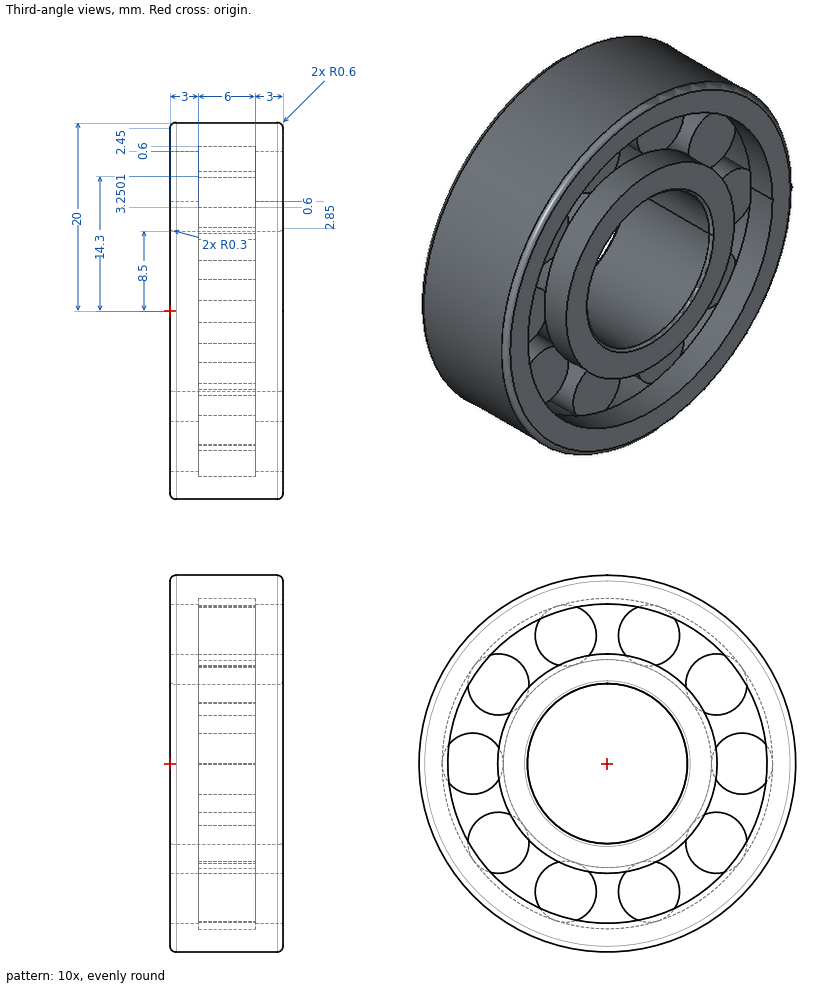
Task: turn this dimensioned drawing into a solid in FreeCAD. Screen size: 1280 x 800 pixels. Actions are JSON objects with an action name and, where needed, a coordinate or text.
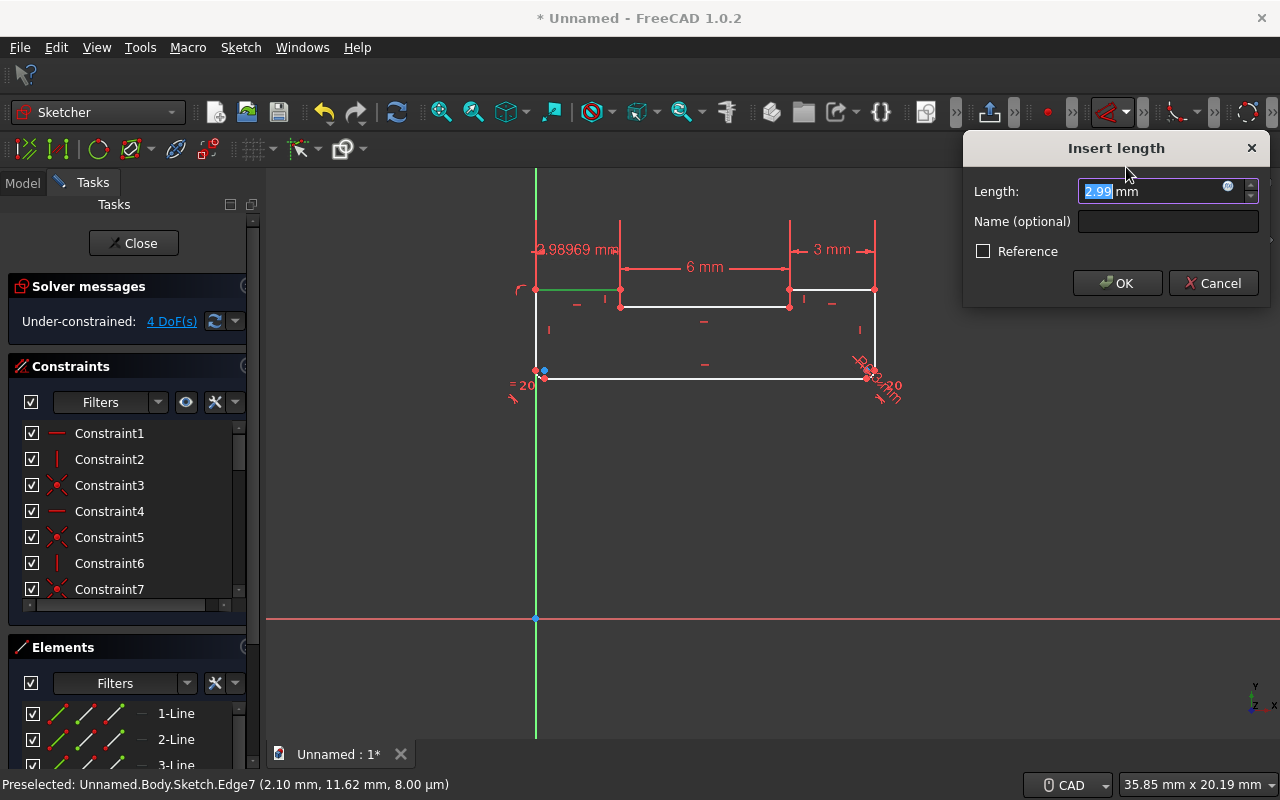
{"action": "type", "text": "3"}
{"action": "key", "text": "Return"}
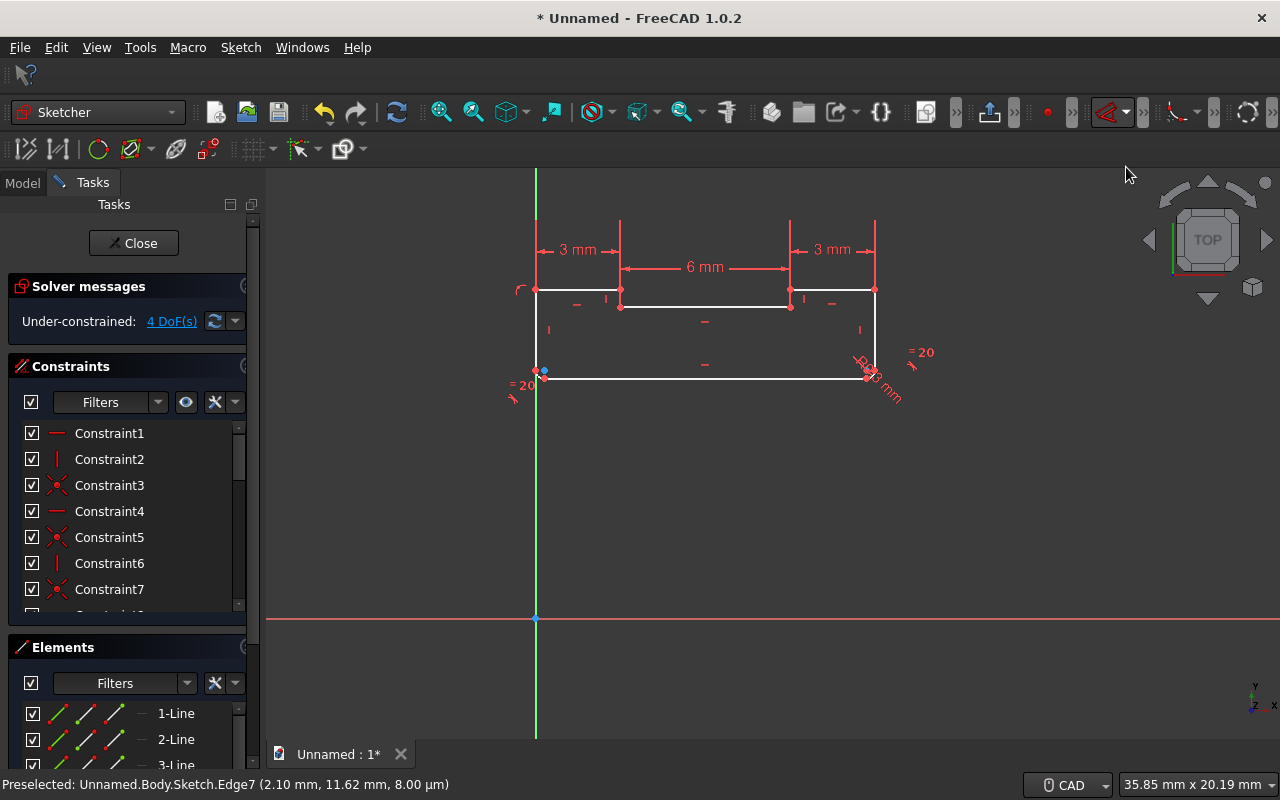
{"action": "scroll", "coordinate": [790, 298], "scroll_direction": "up", "scroll_amount": 5}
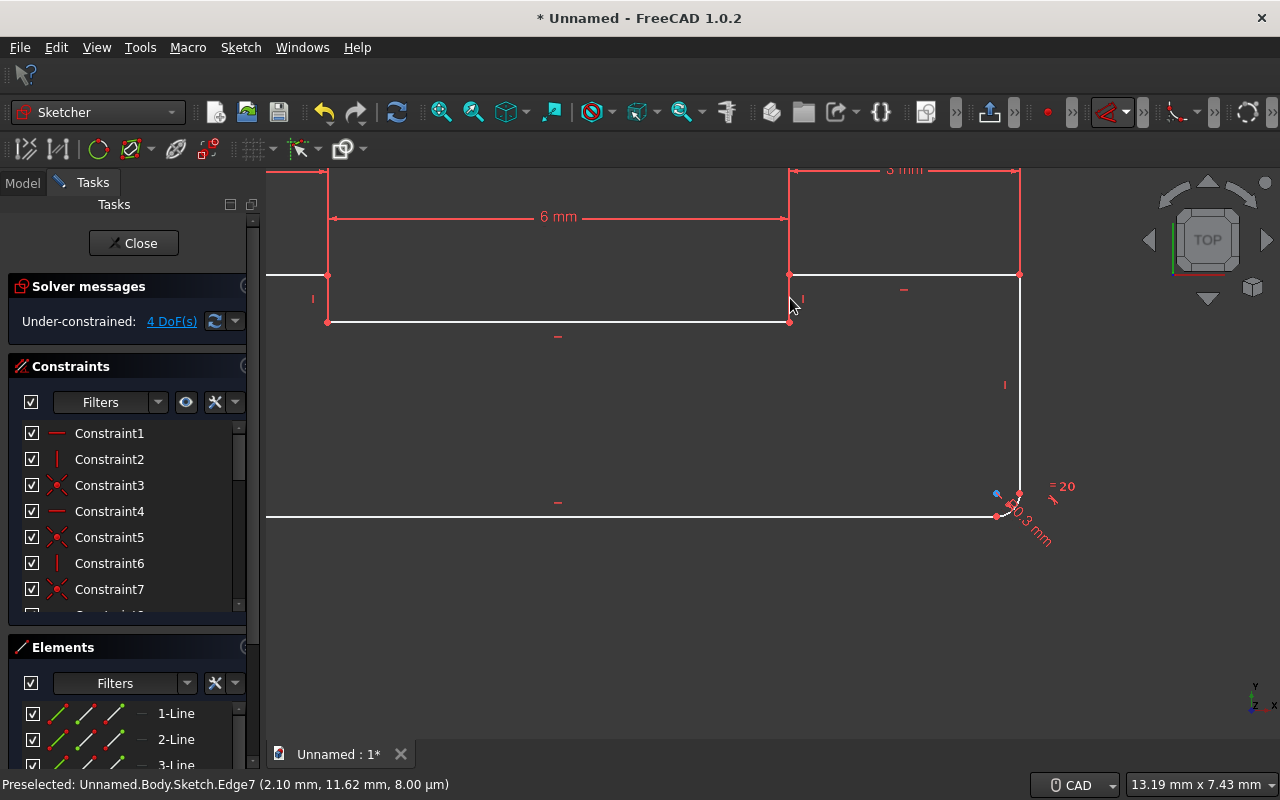
{"action": "left_click", "coordinate": [789, 298]}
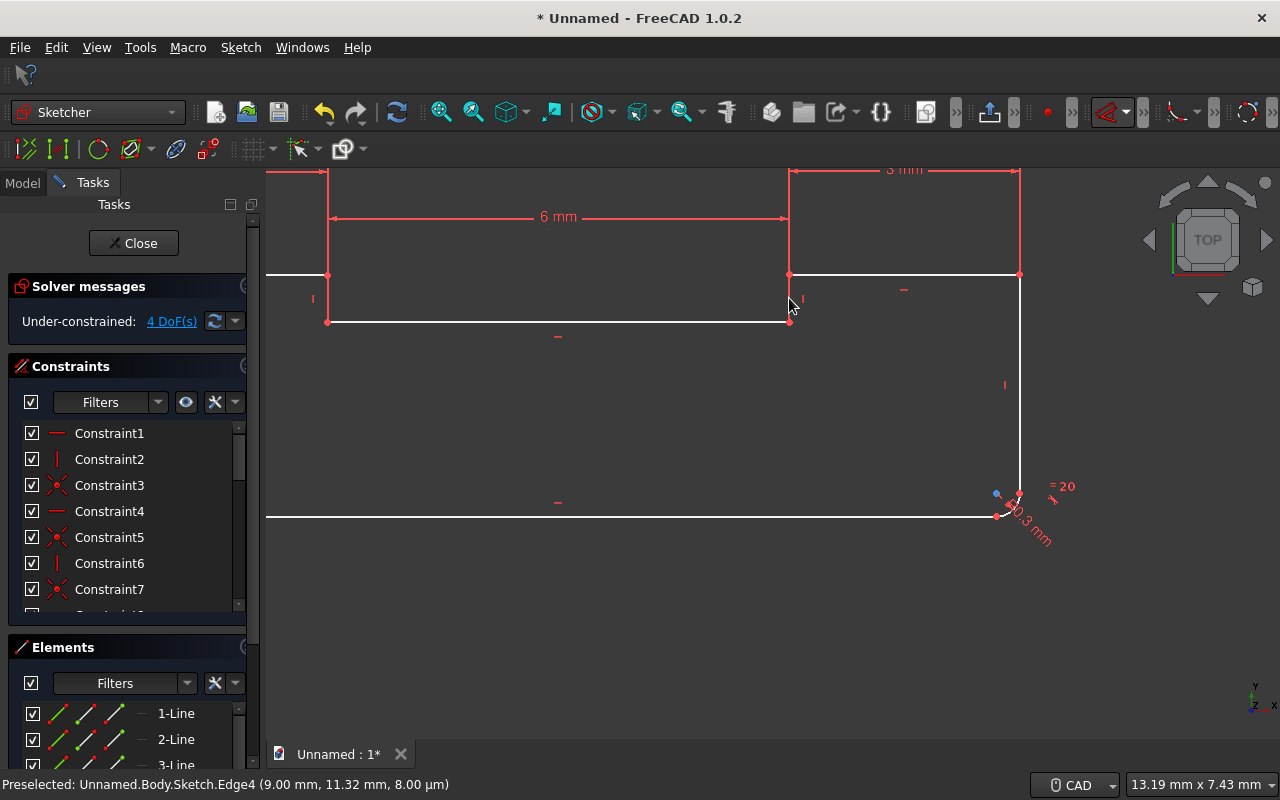
{"action": "left_click", "coordinate": [1128, 112]}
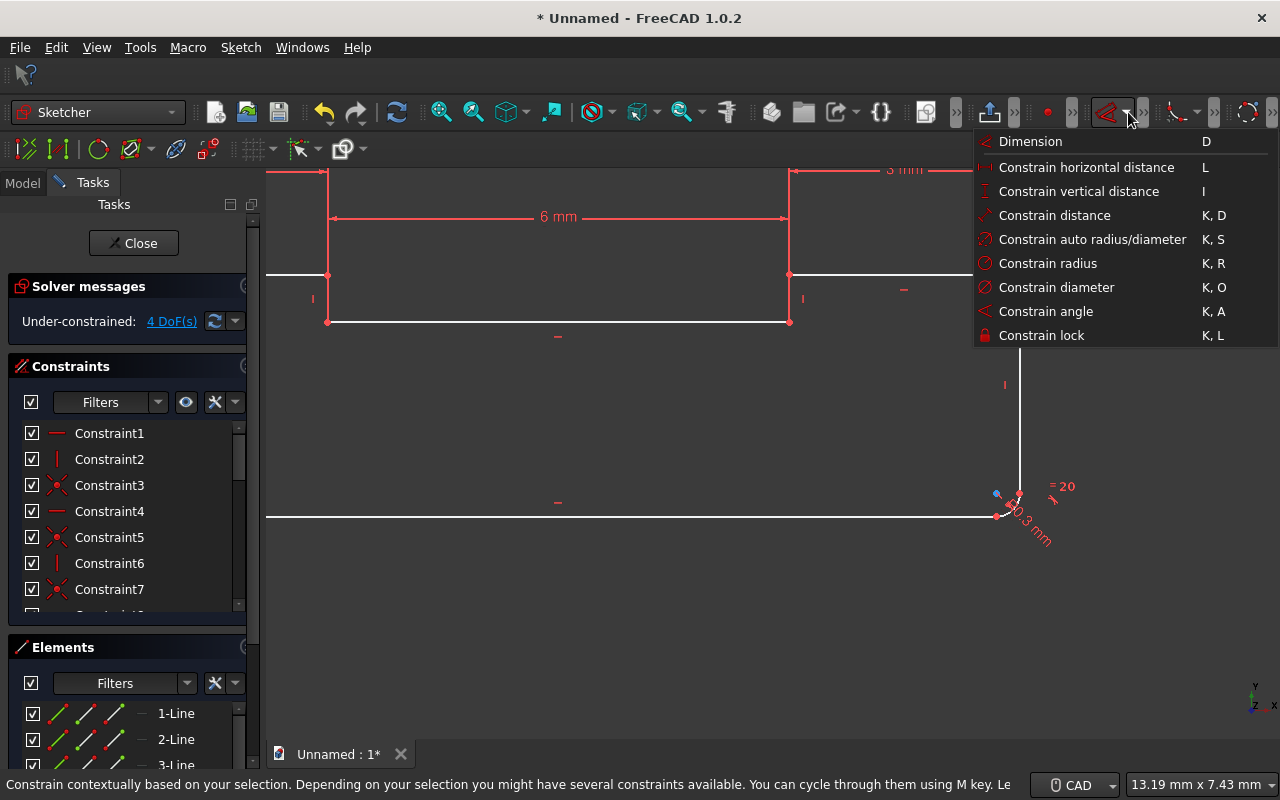
{"action": "left_click", "coordinate": [1126, 191]}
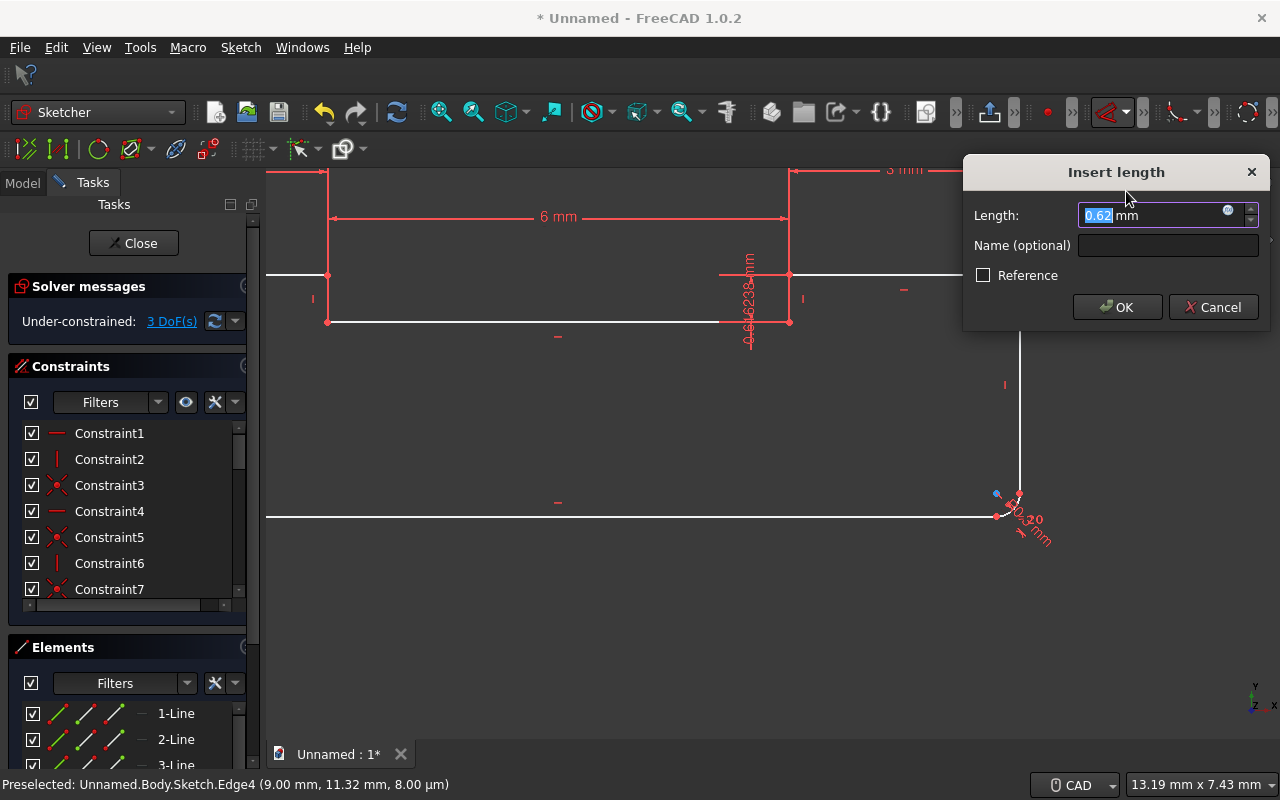
{"action": "type", "text": "0.6"}
{"action": "key", "text": "Return"}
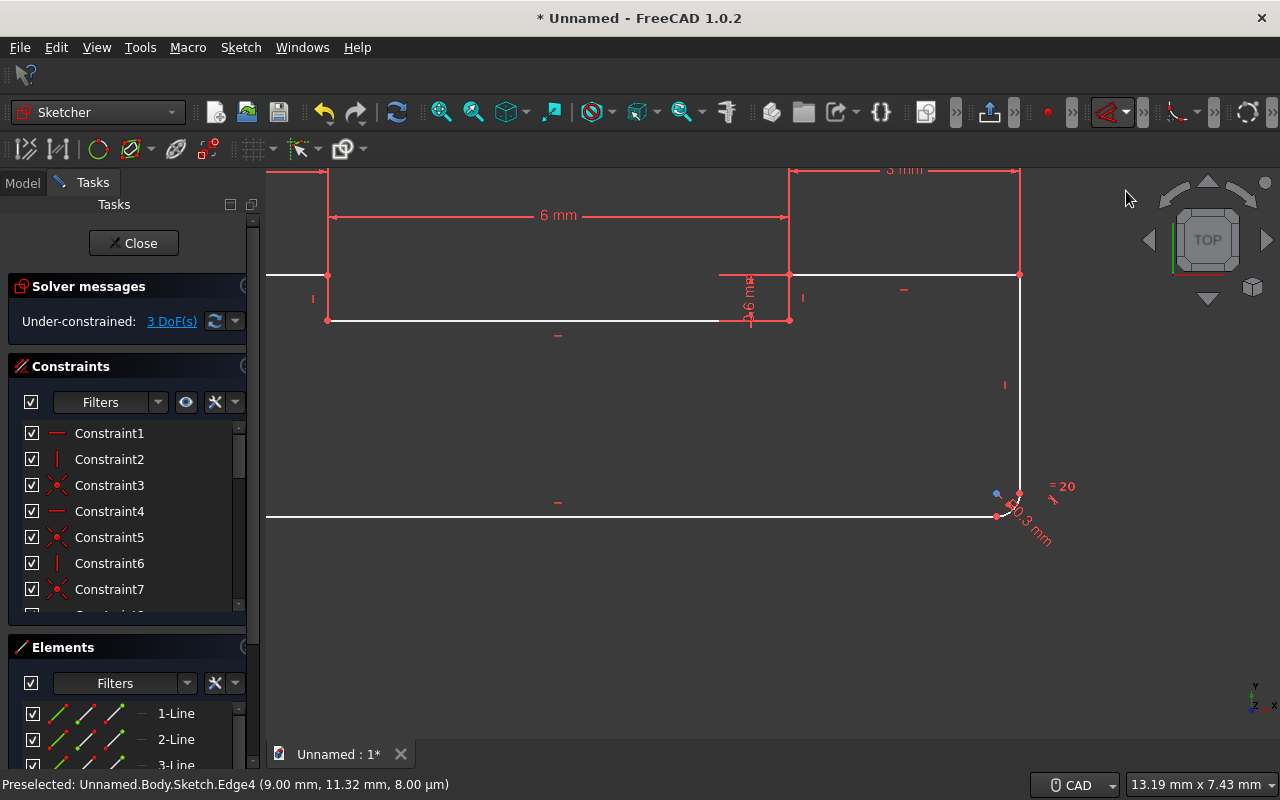
{"action": "left_click", "coordinate": [328, 307]}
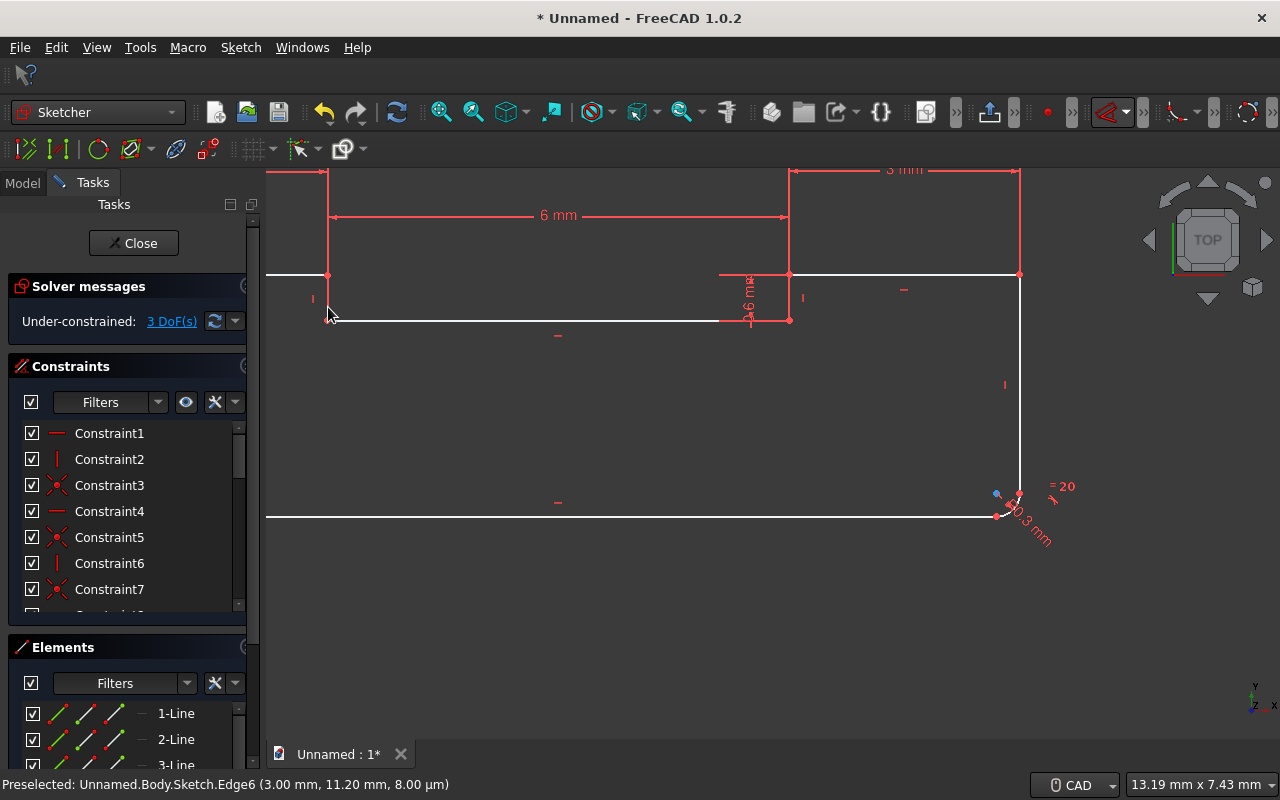
{"action": "left_click", "coordinate": [1128, 112]}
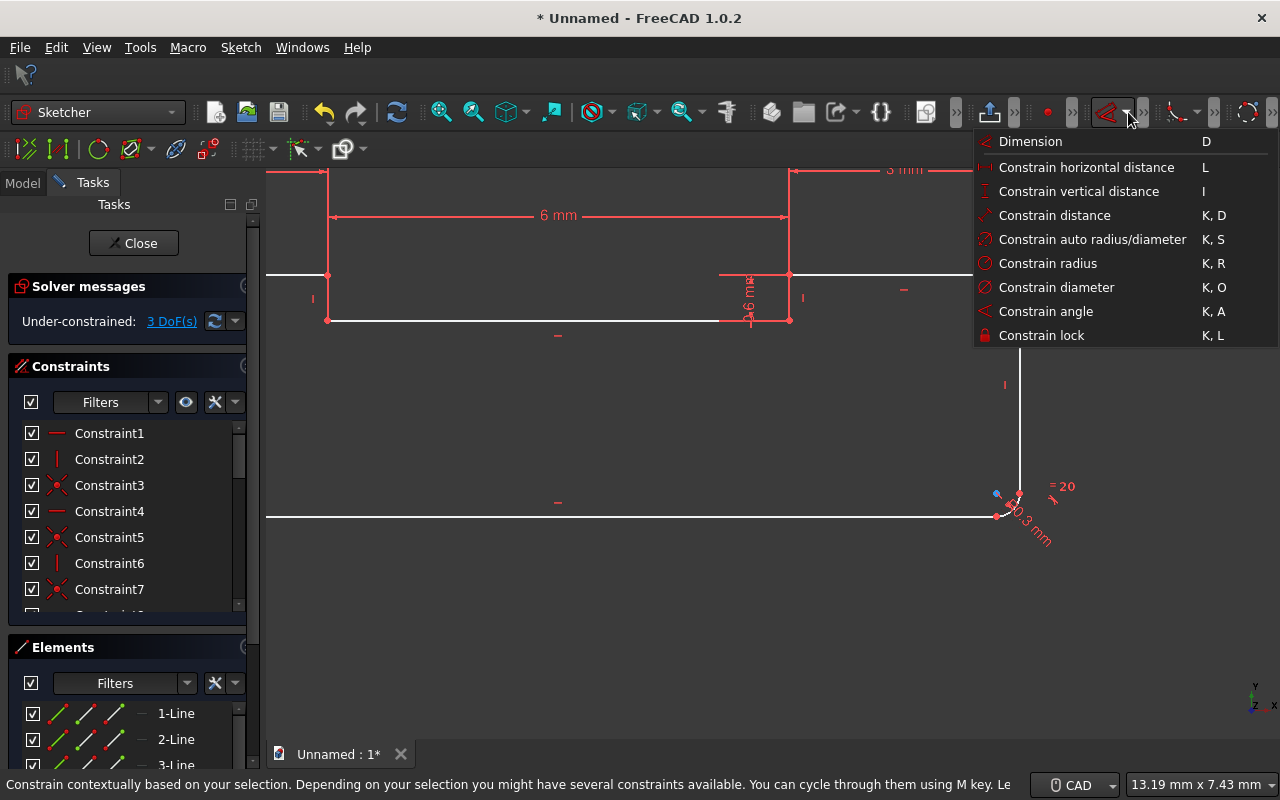
{"action": "left_click", "coordinate": [1126, 191]}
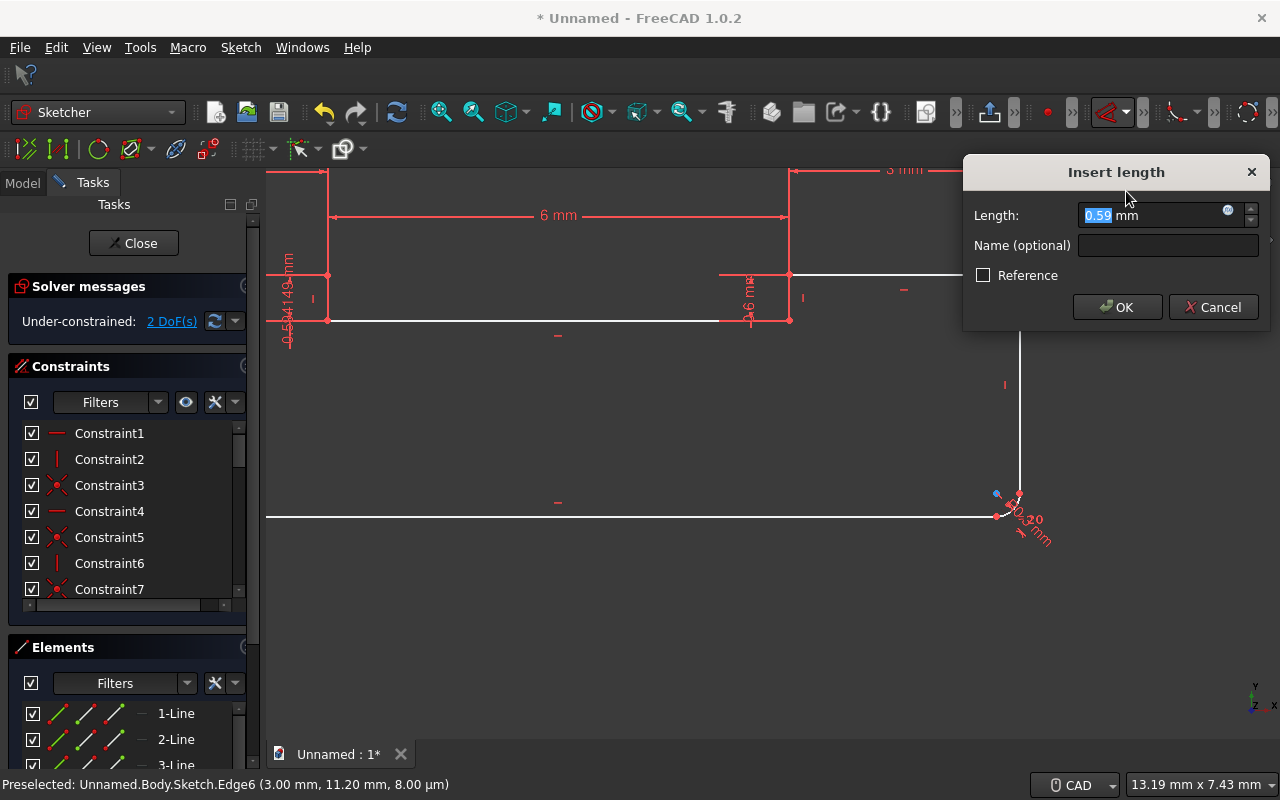
{"action": "type", "text": "0.6"}
{"action": "key", "text": "Return"}